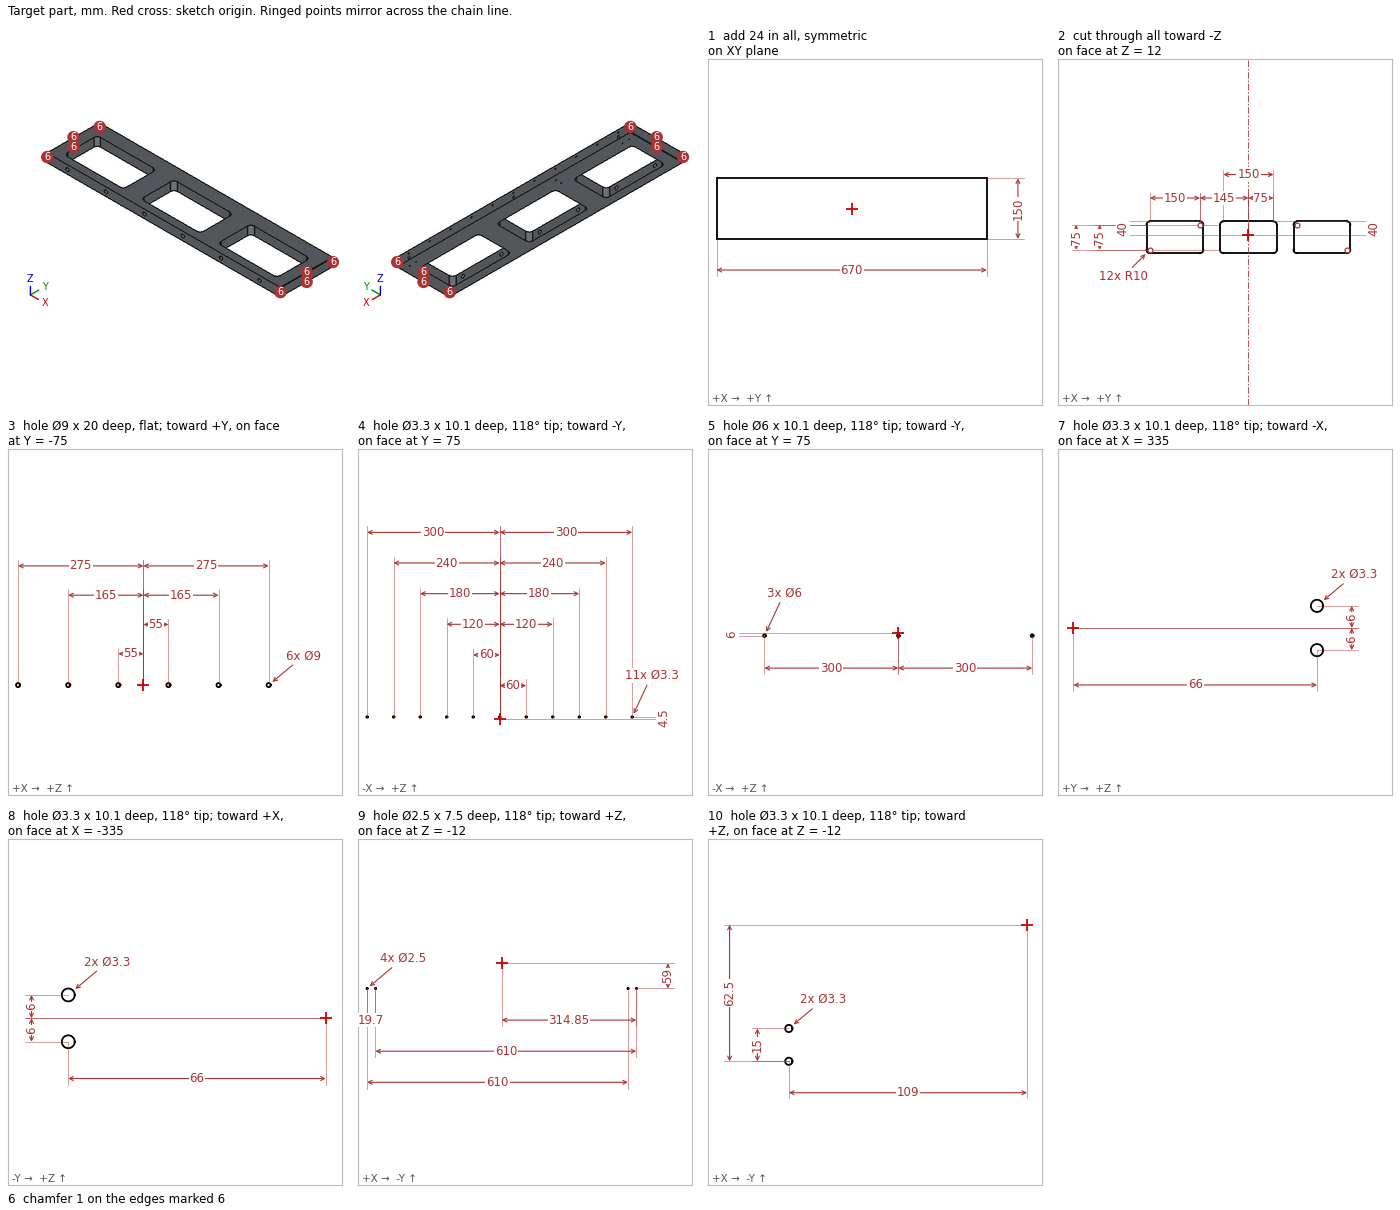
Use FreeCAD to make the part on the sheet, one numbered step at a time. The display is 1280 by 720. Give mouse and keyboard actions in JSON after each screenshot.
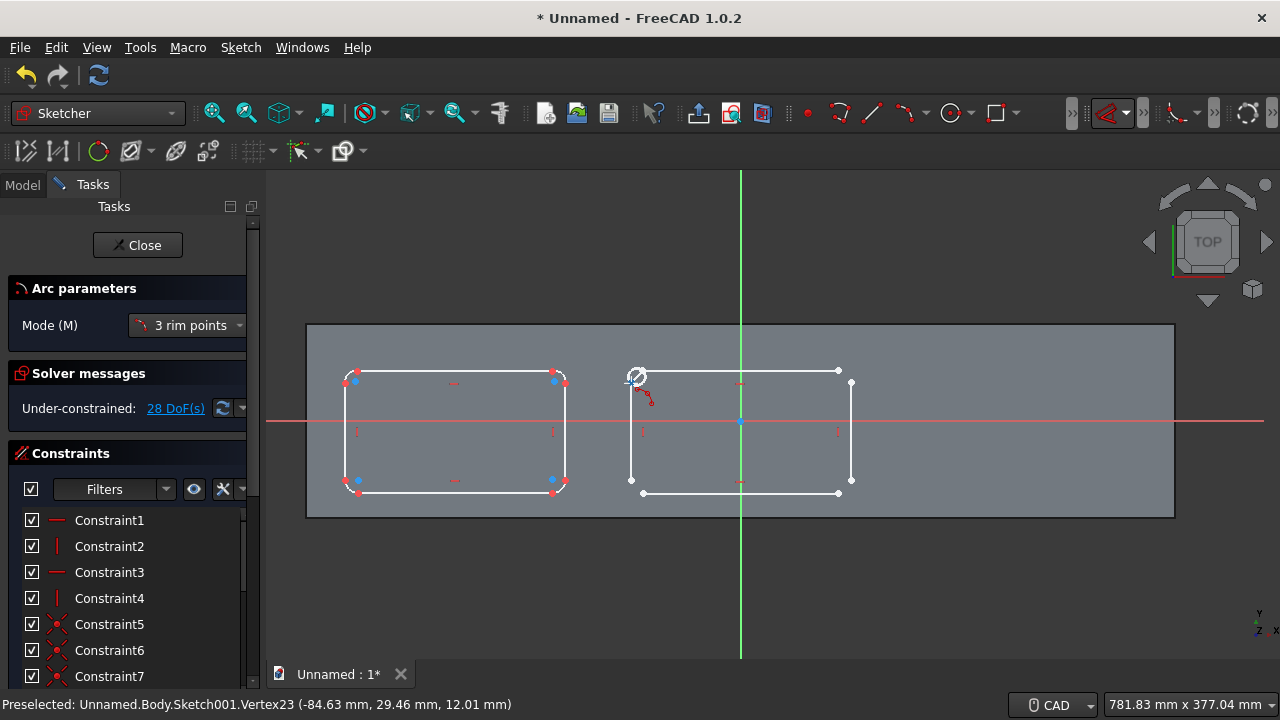
{"action": "scroll", "coordinate": [634, 373], "scroll_direction": "up", "scroll_amount": 8}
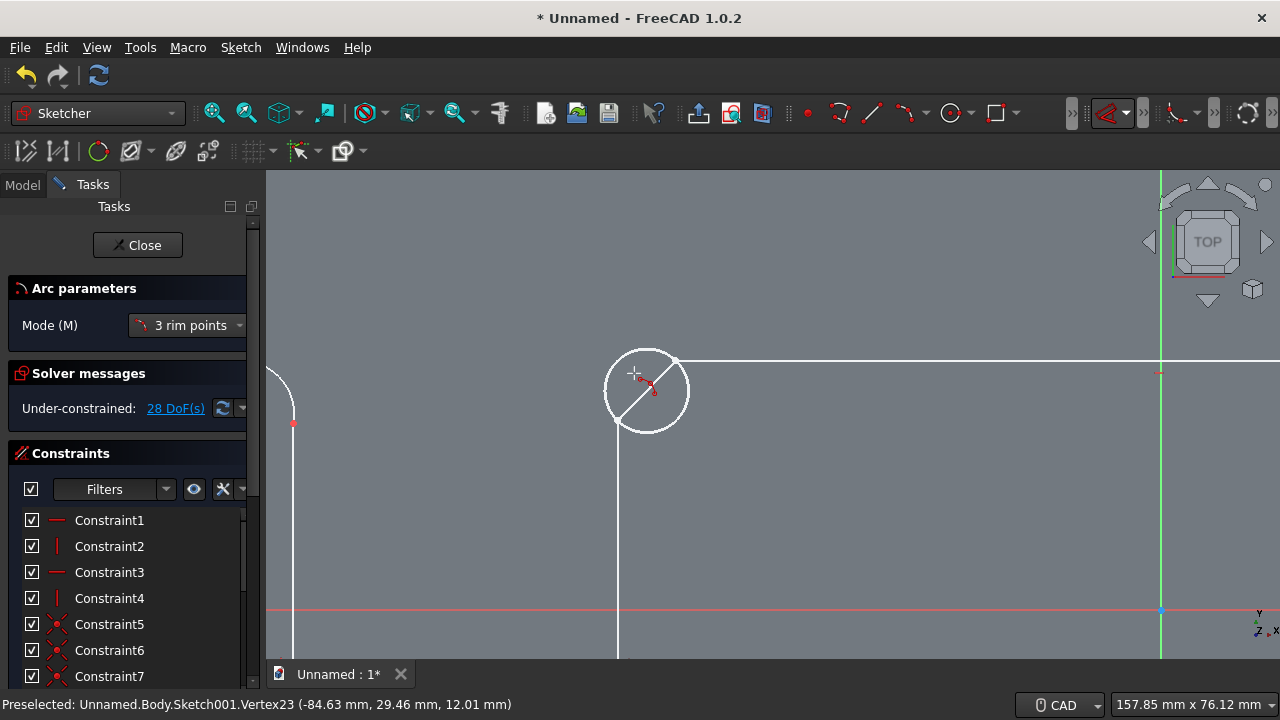
{"action": "left_click", "coordinate": [634, 372]}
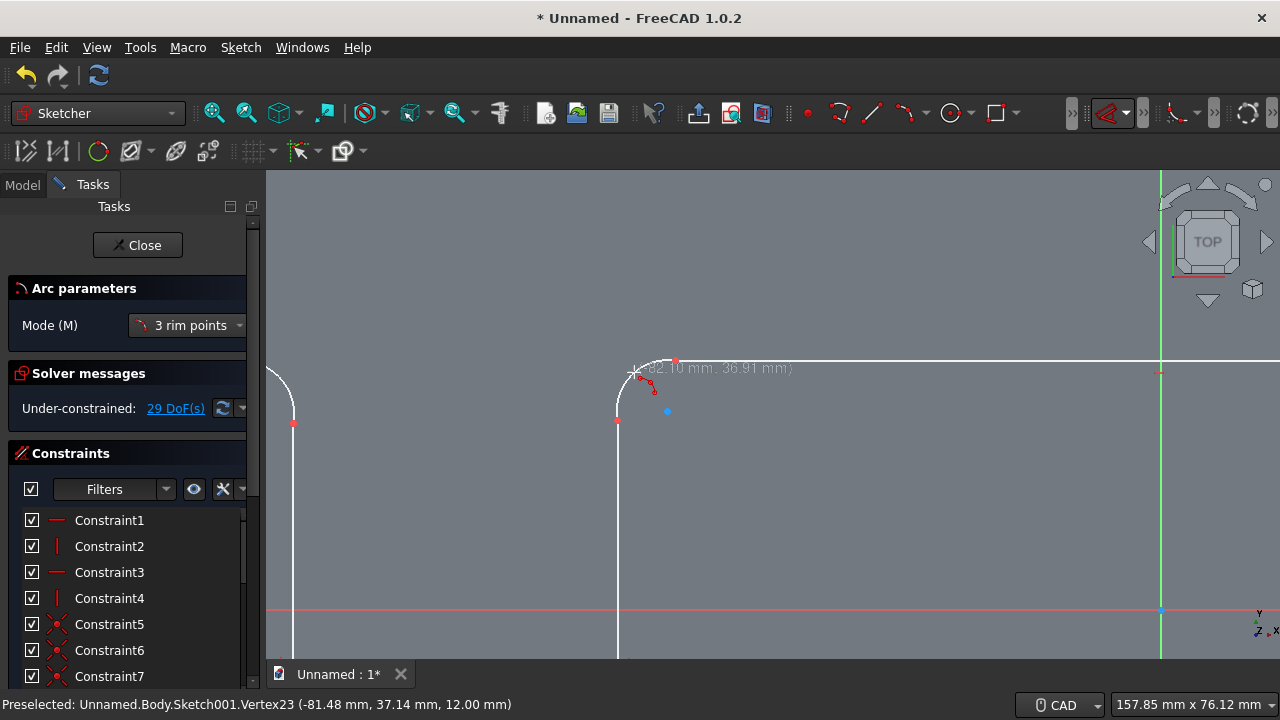
{"action": "scroll", "coordinate": [633, 376], "scroll_direction": "down", "scroll_amount": 10}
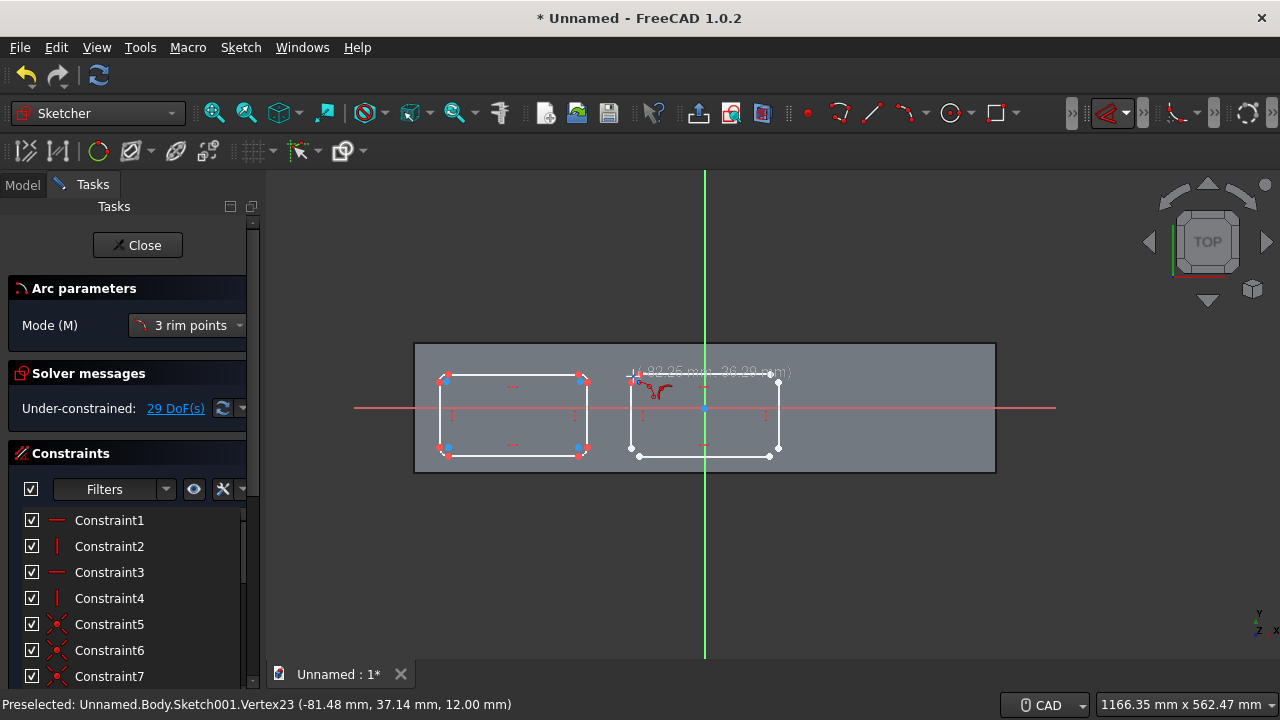
{"action": "scroll", "coordinate": [631, 447], "scroll_direction": "up", "scroll_amount": 2}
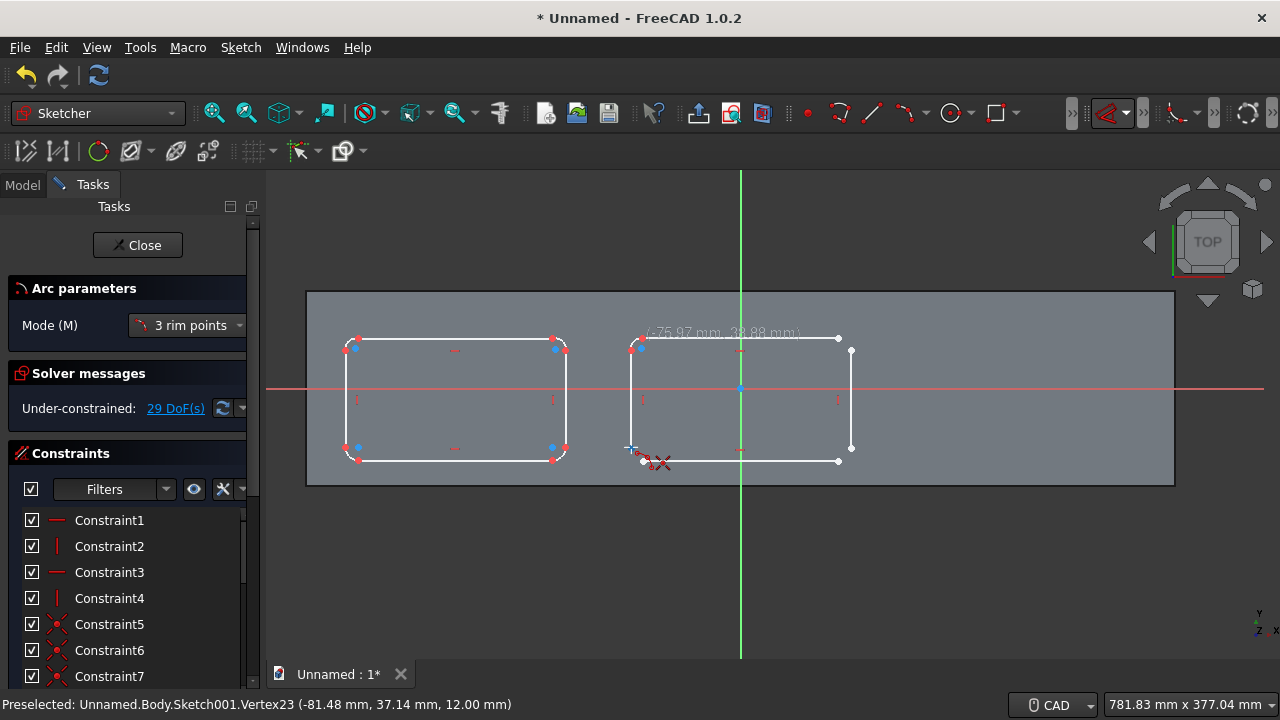
{"action": "left_click", "coordinate": [631, 448]}
{"action": "left_click", "coordinate": [643, 461]}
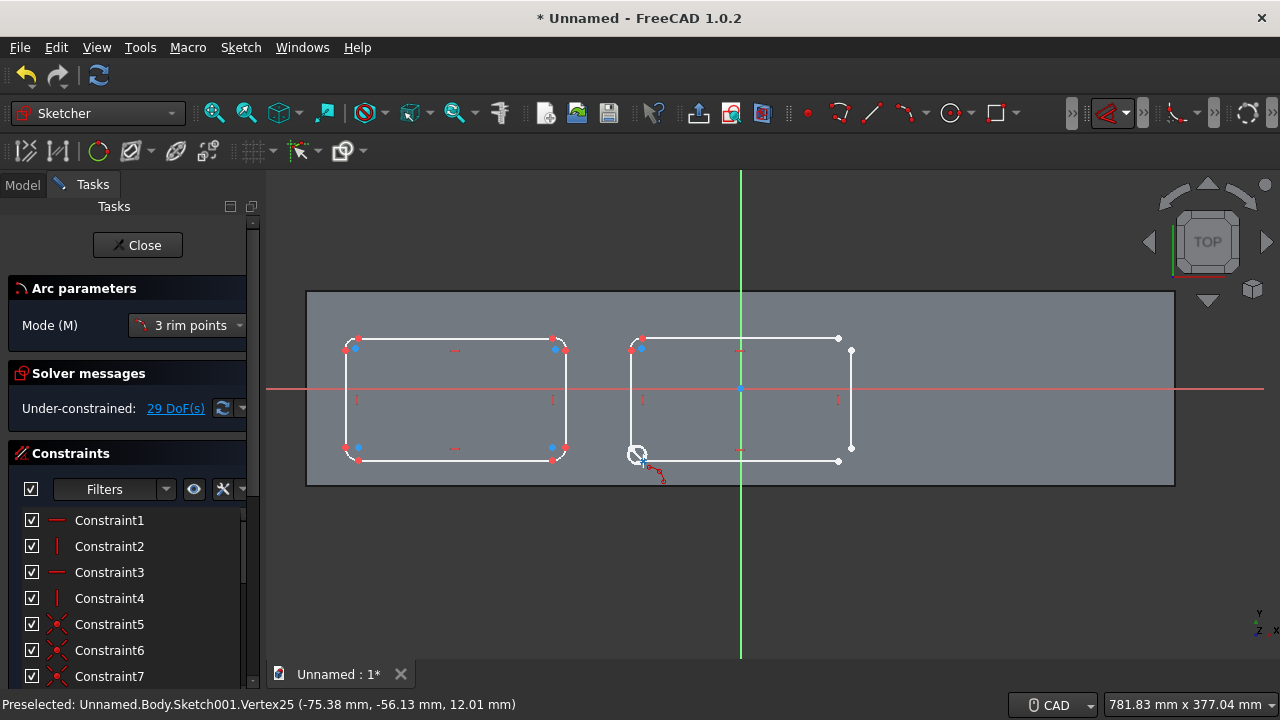
{"action": "scroll", "coordinate": [635, 456], "scroll_direction": "up", "scroll_amount": 8}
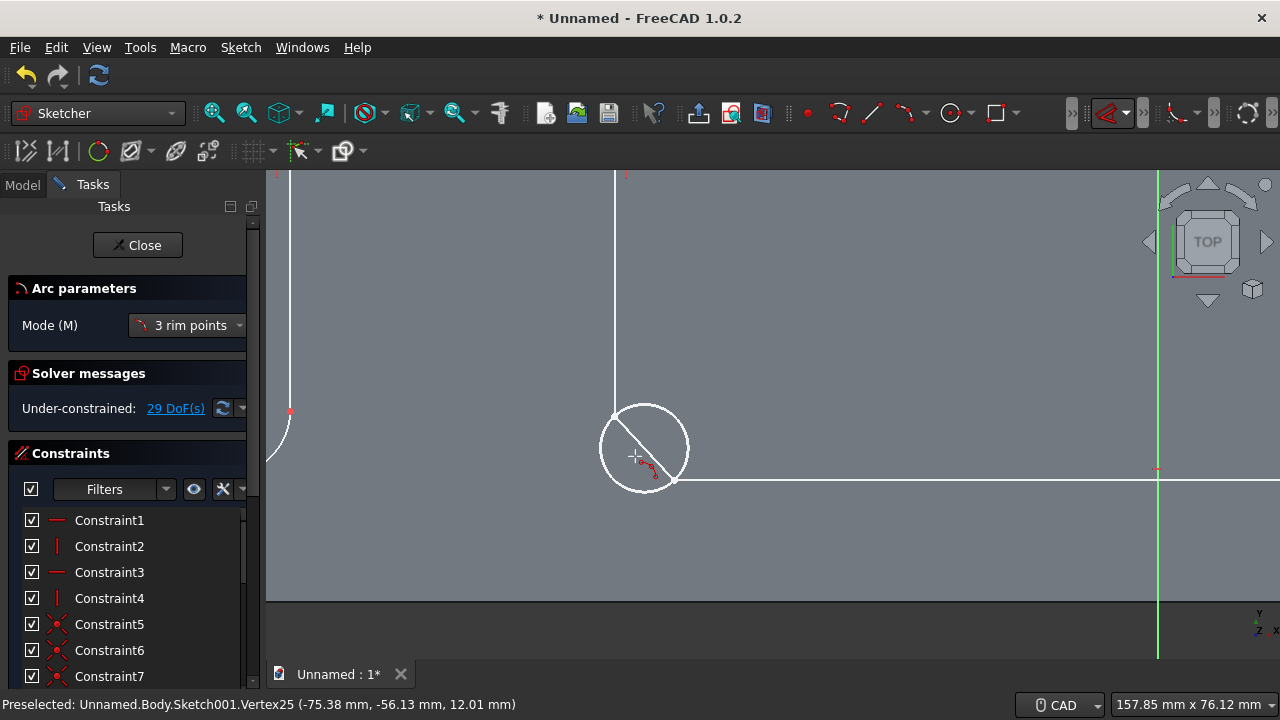
{"action": "left_click", "coordinate": [631, 454]}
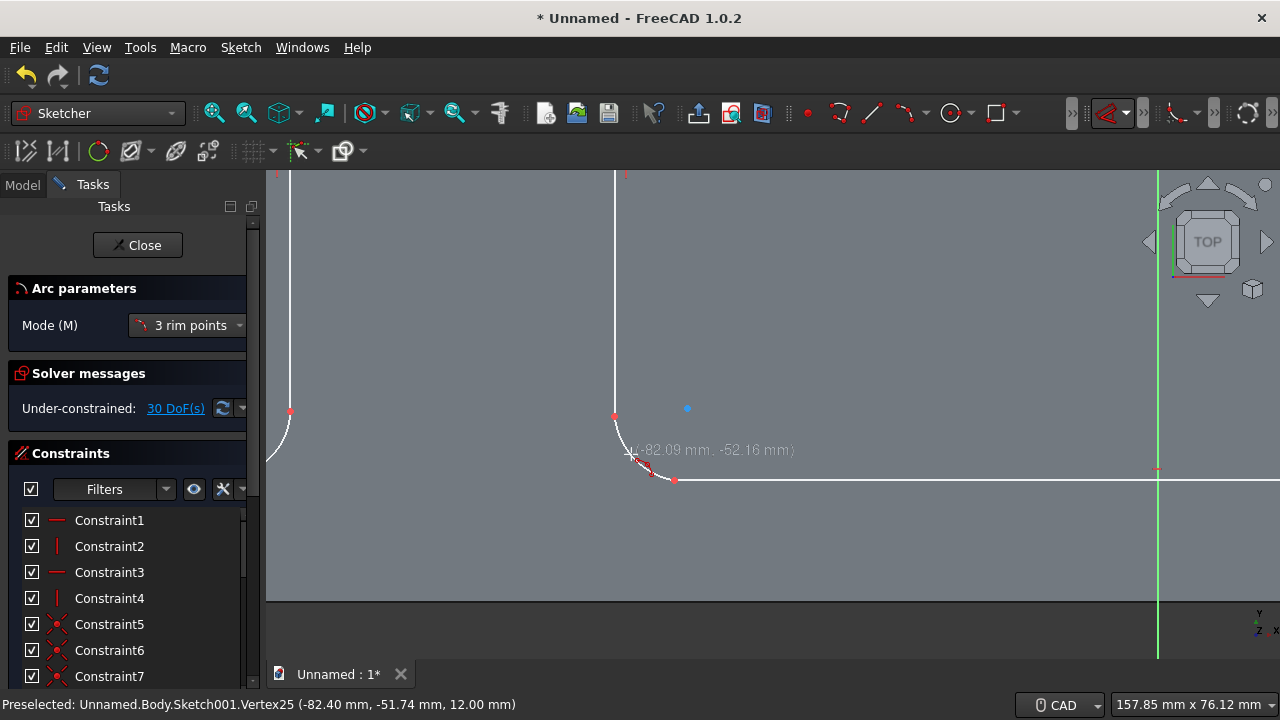
{"action": "scroll", "coordinate": [633, 453], "scroll_direction": "down", "scroll_amount": 10}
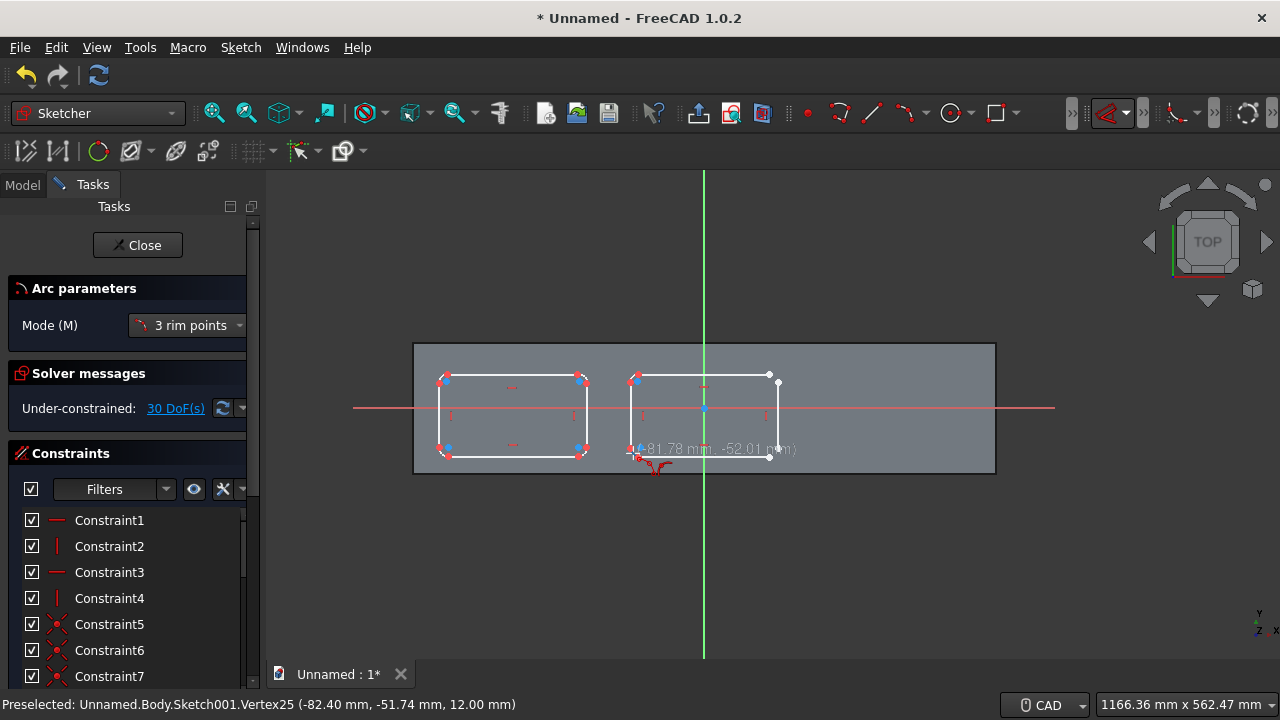
{"action": "scroll", "coordinate": [770, 456], "scroll_direction": "up", "scroll_amount": 2}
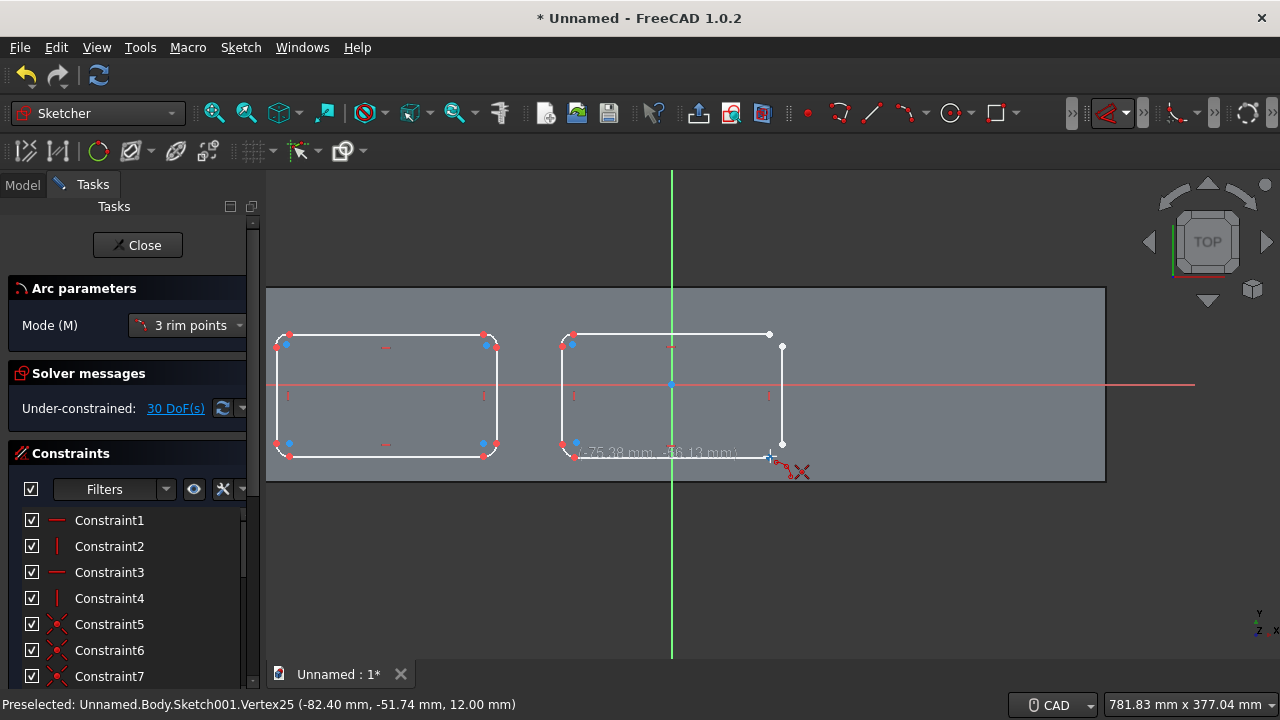
{"action": "left_click", "coordinate": [769, 458]}
{"action": "left_click", "coordinate": [782, 445]}